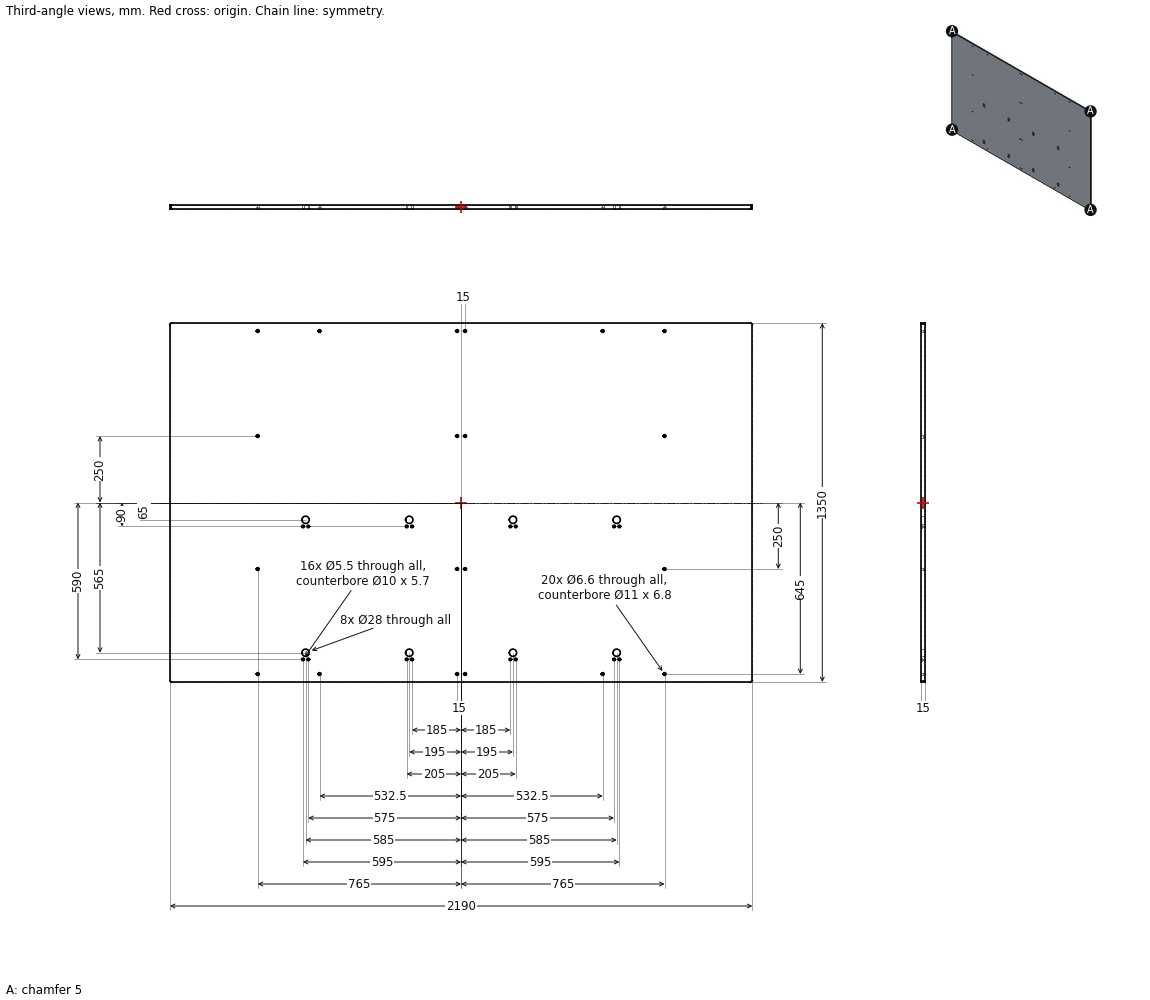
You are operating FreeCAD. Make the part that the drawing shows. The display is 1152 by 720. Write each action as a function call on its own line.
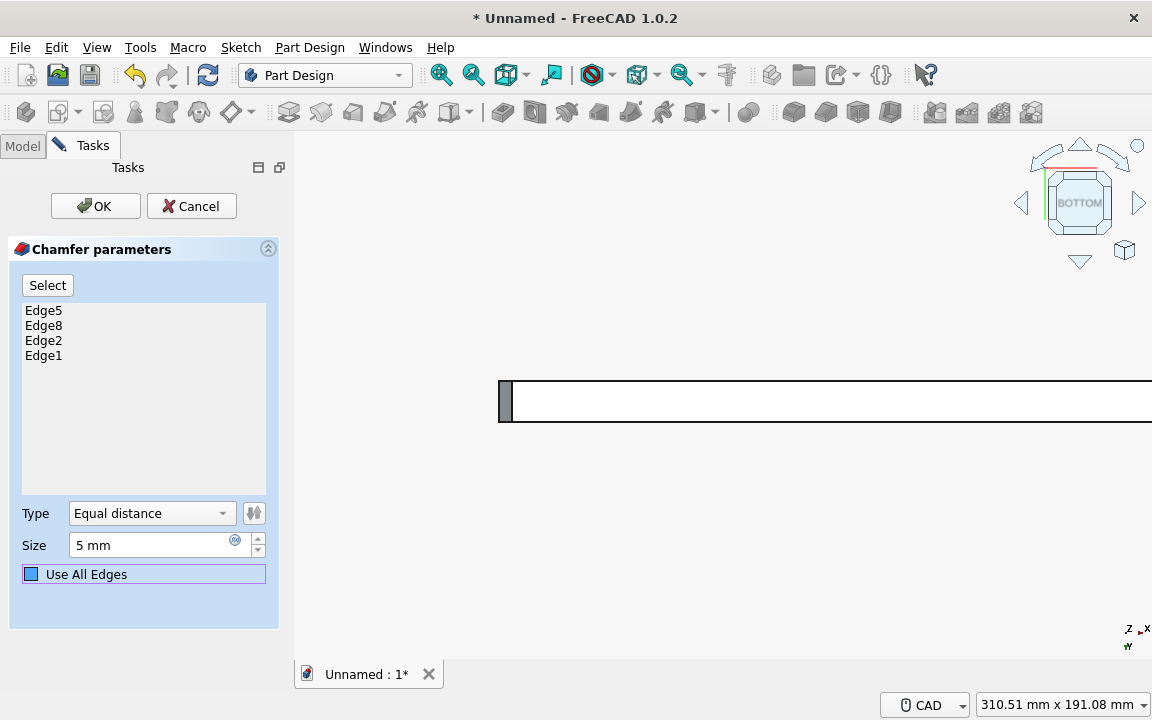
click(96, 206)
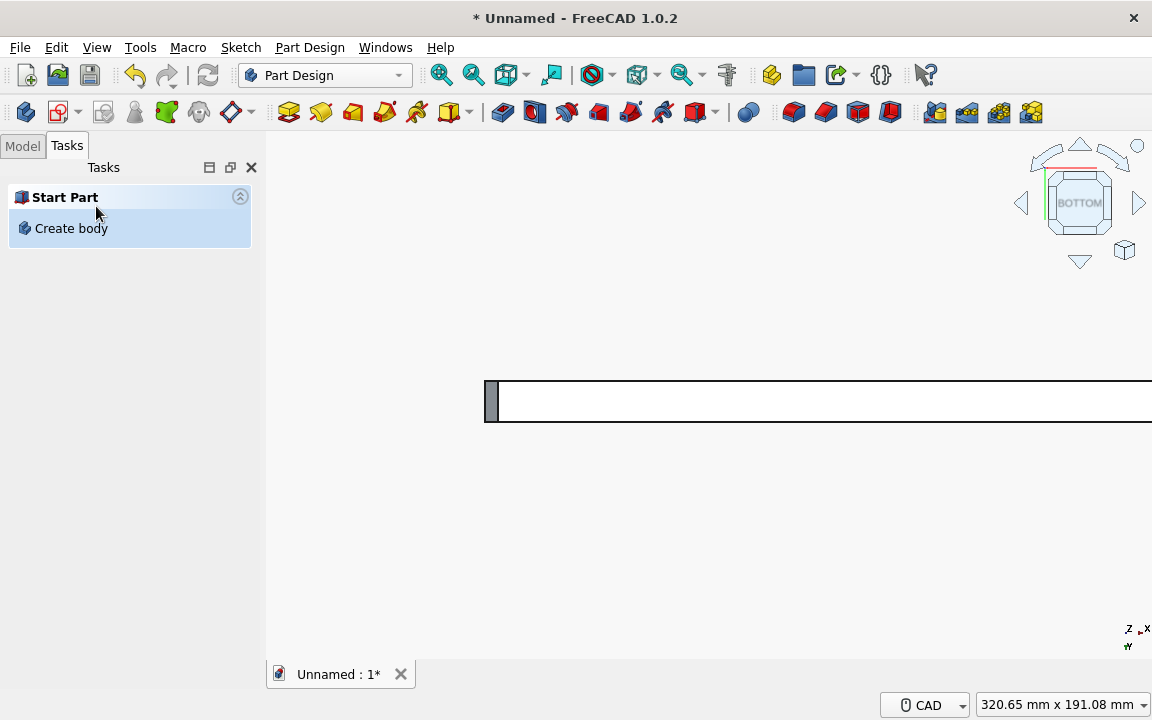
key(v)
key(f)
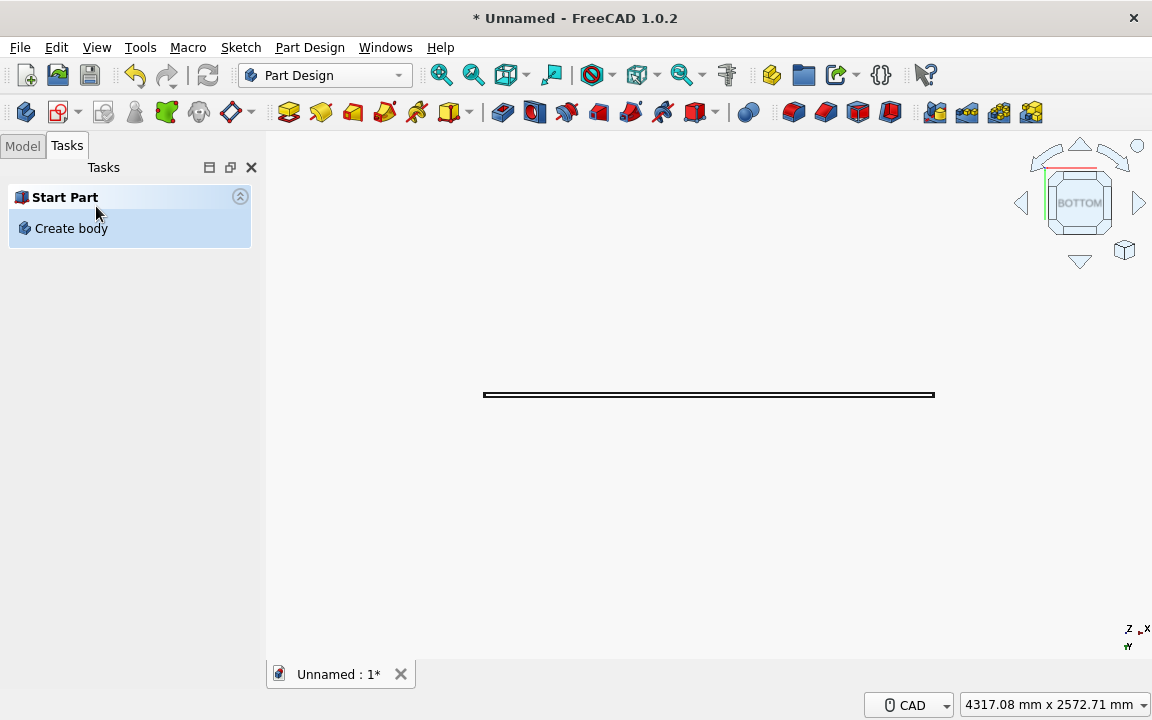
key(4)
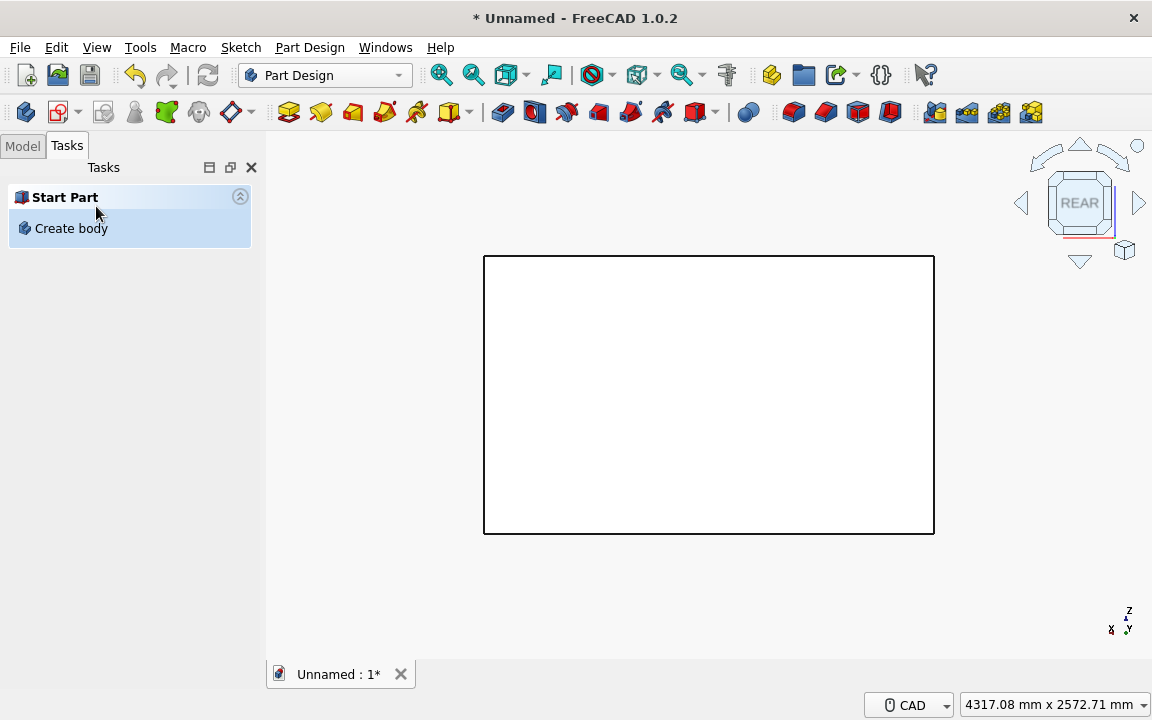
click(645, 394)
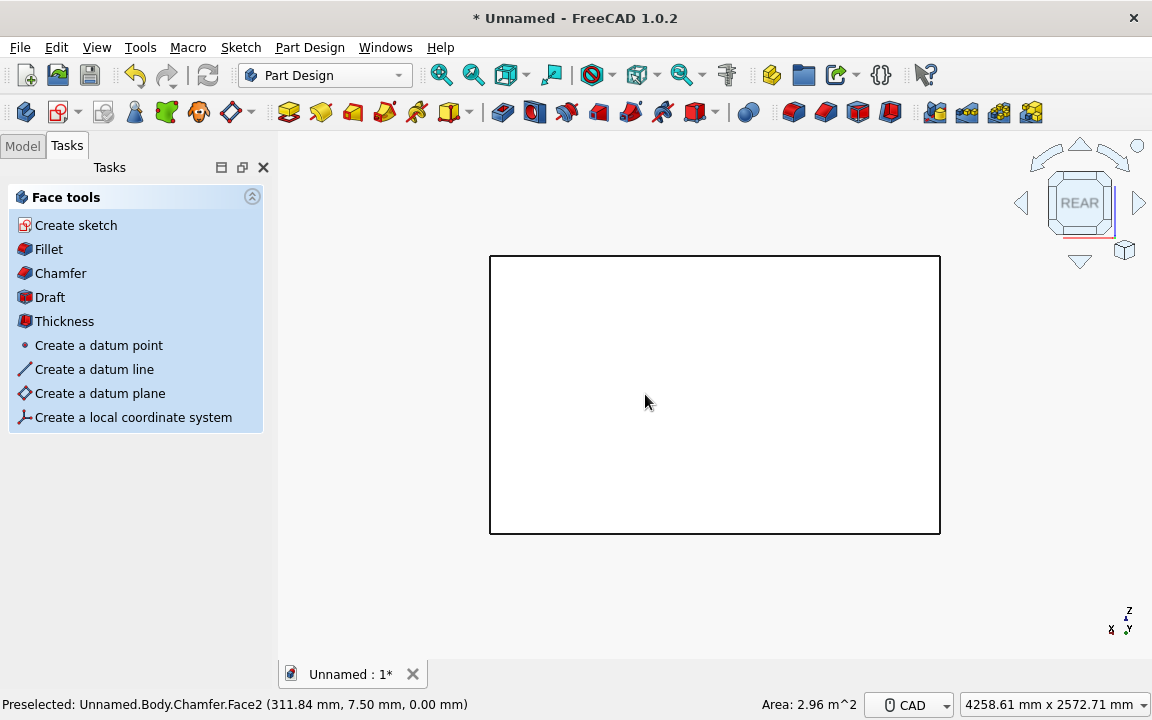
click(58, 112)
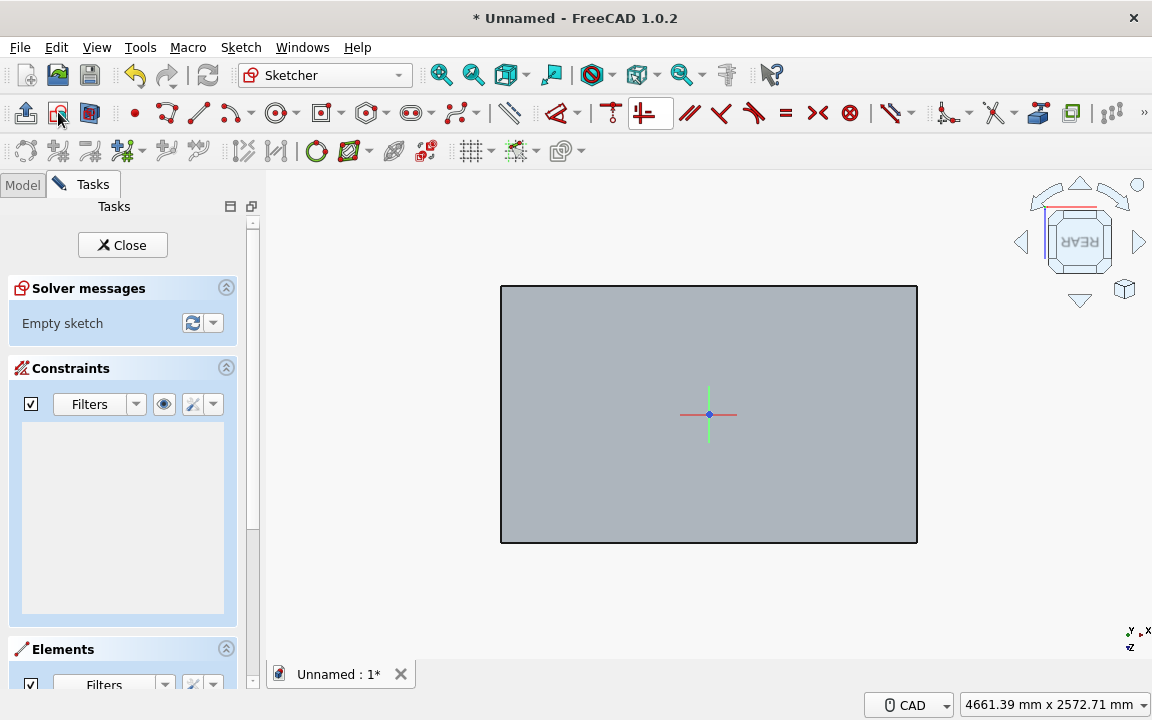
scroll(765, 315, up, 4)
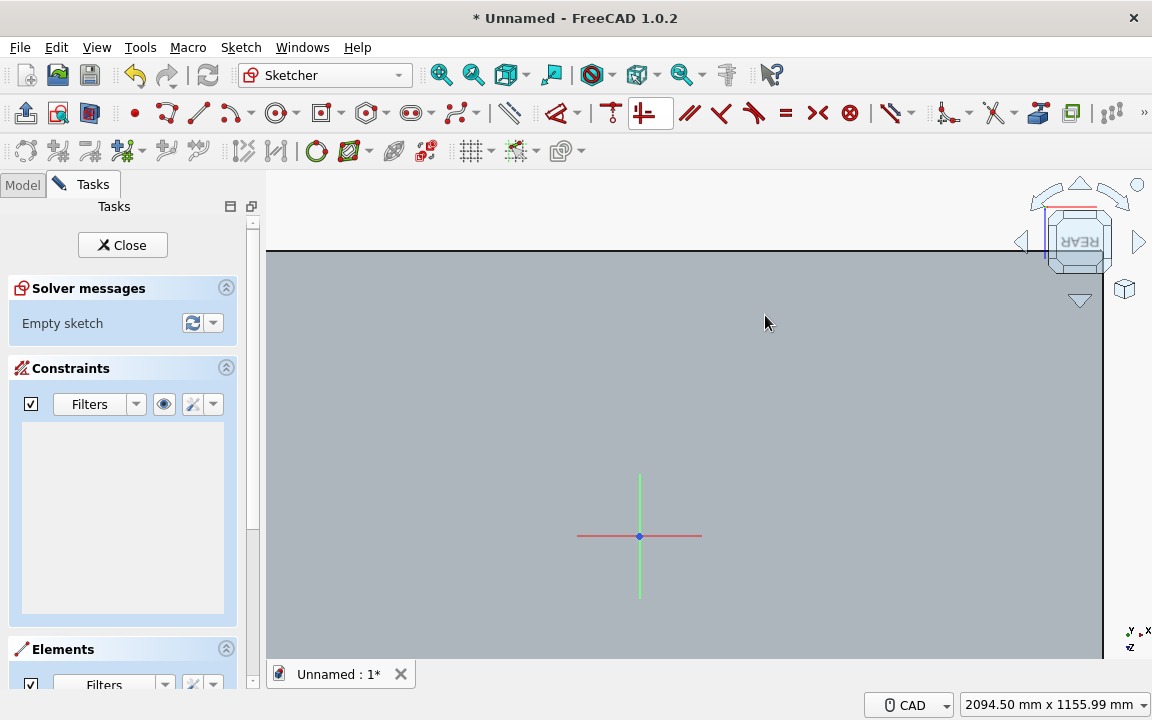
key(g)
key(c)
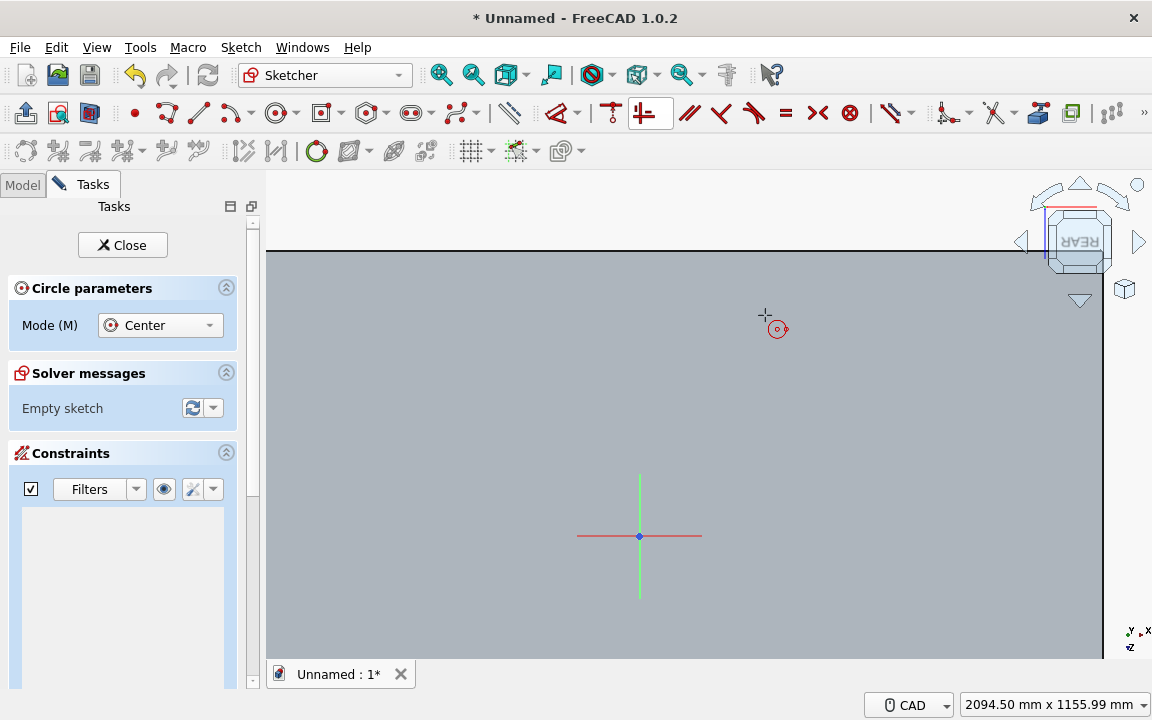
scroll(392, 297, up, 7)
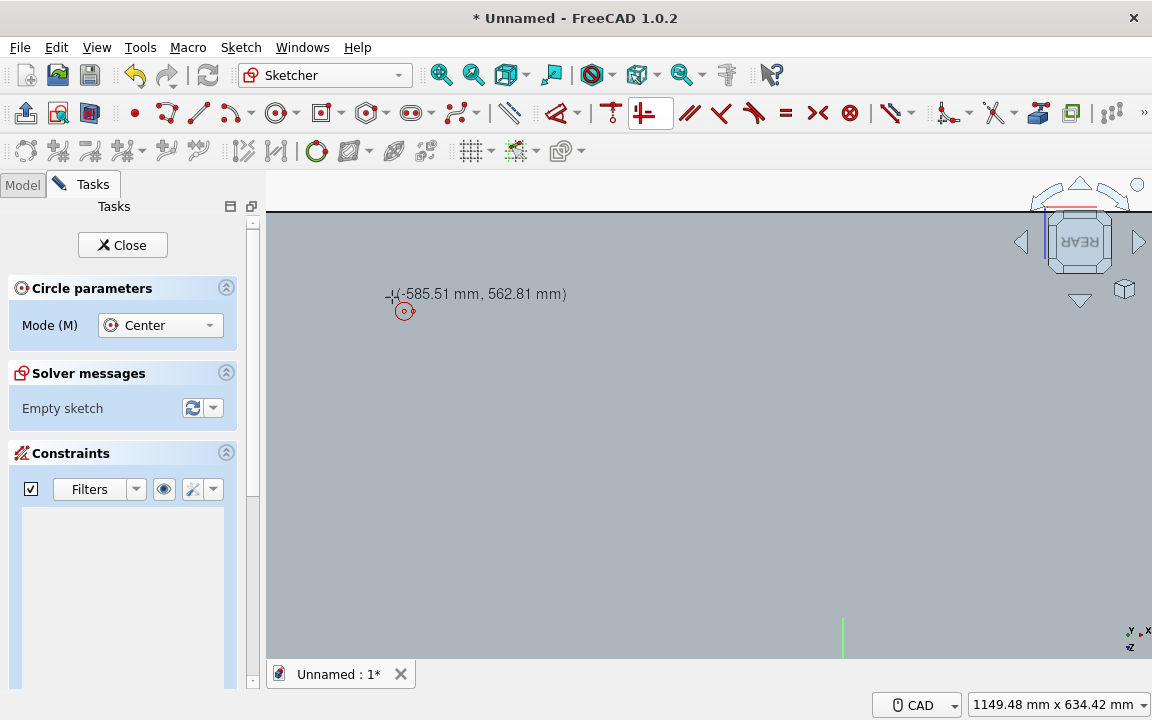
scroll(393, 298, down, 7)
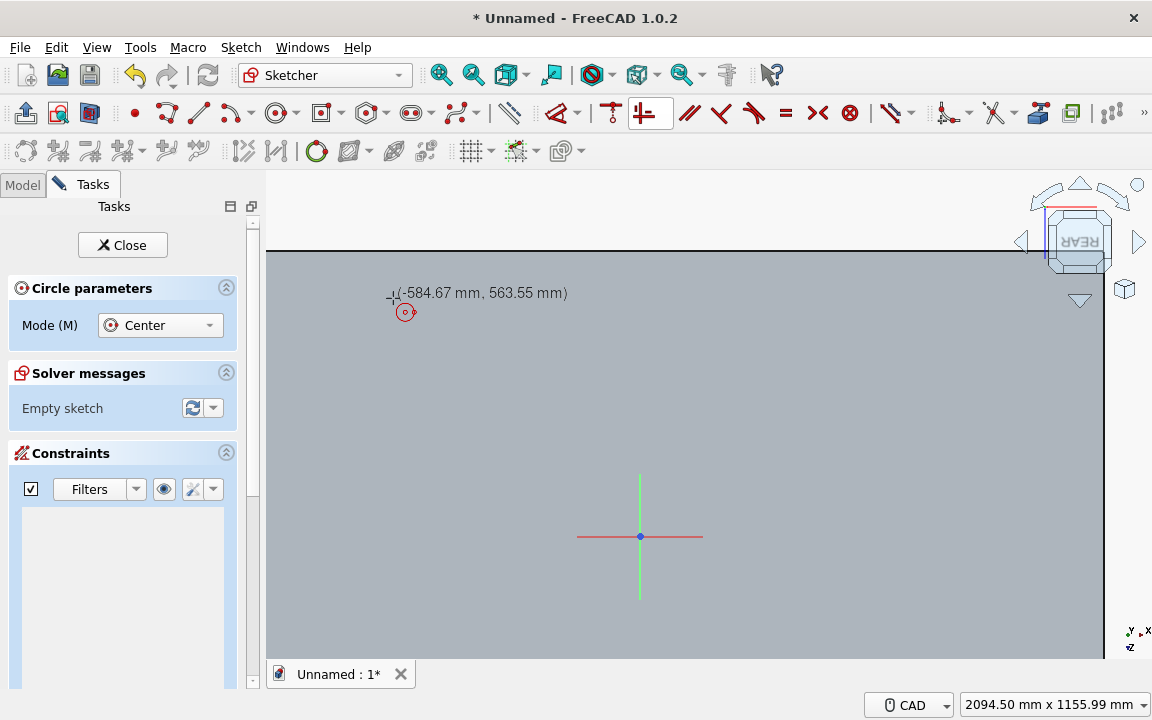
click(393, 298)
move(397, 294)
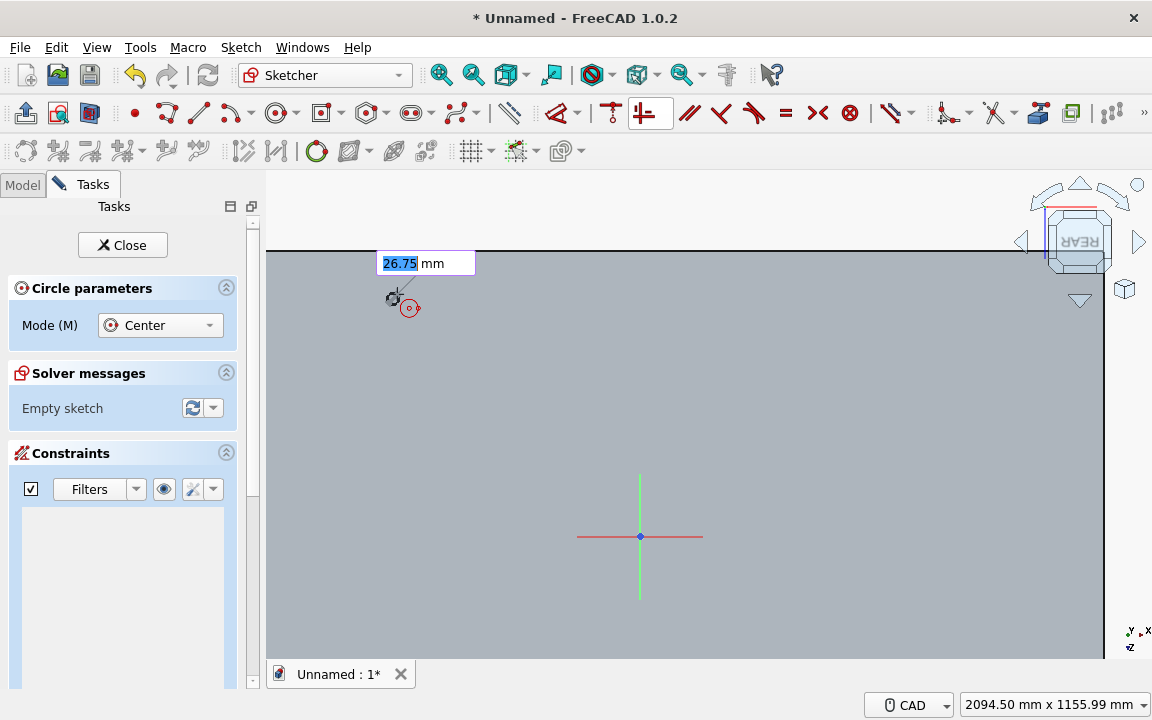
text(28)
key(Return)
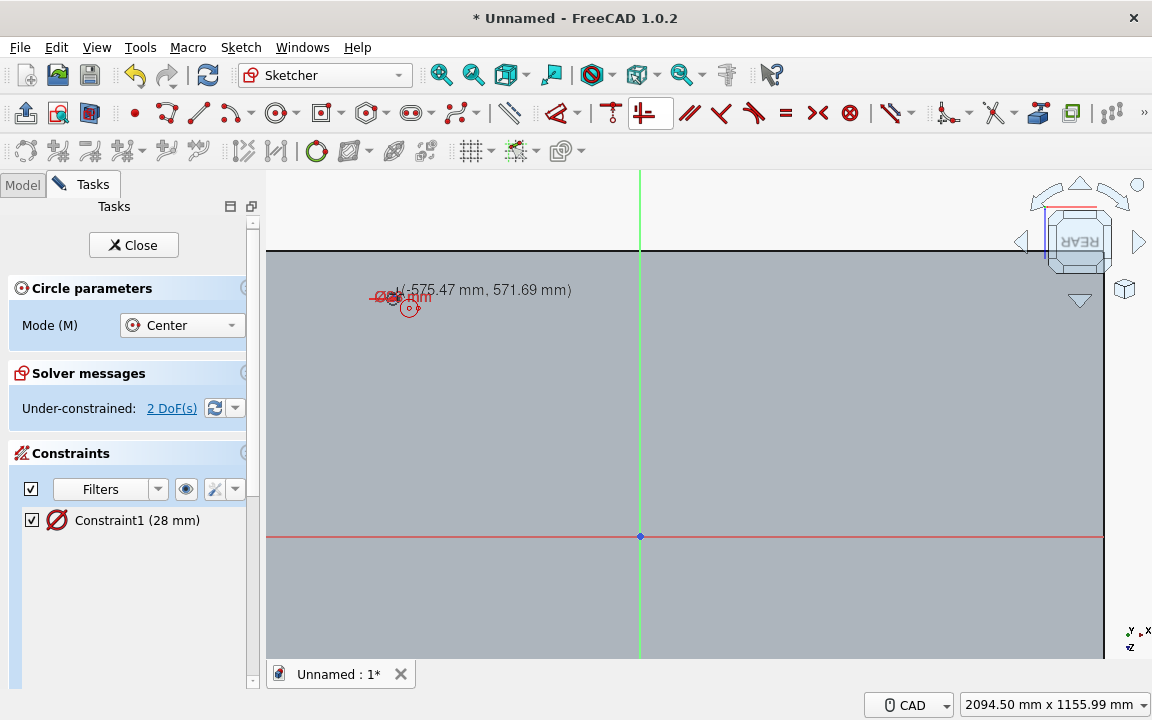
scroll(558, 298, up, 7)